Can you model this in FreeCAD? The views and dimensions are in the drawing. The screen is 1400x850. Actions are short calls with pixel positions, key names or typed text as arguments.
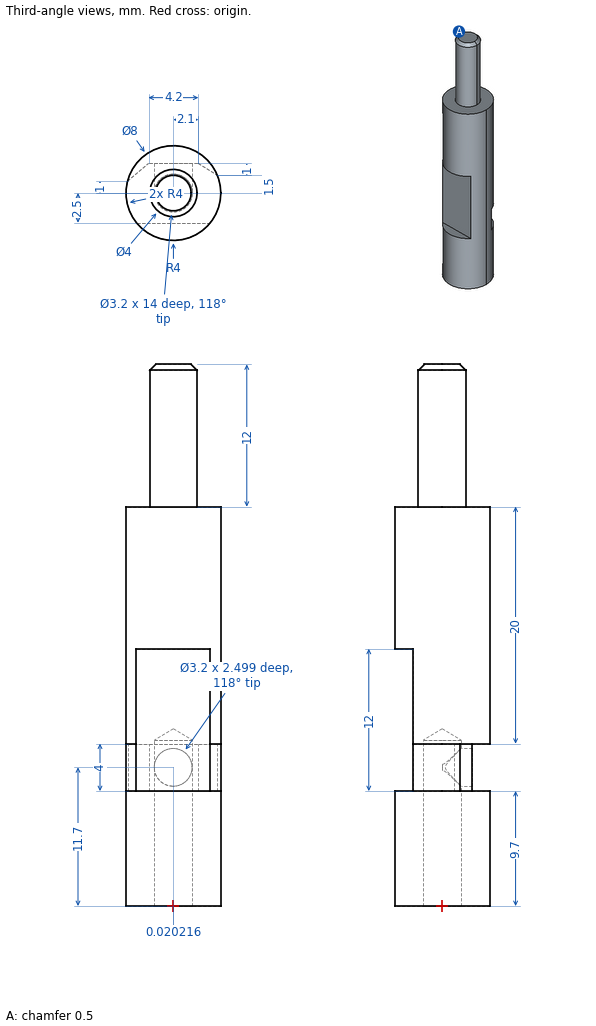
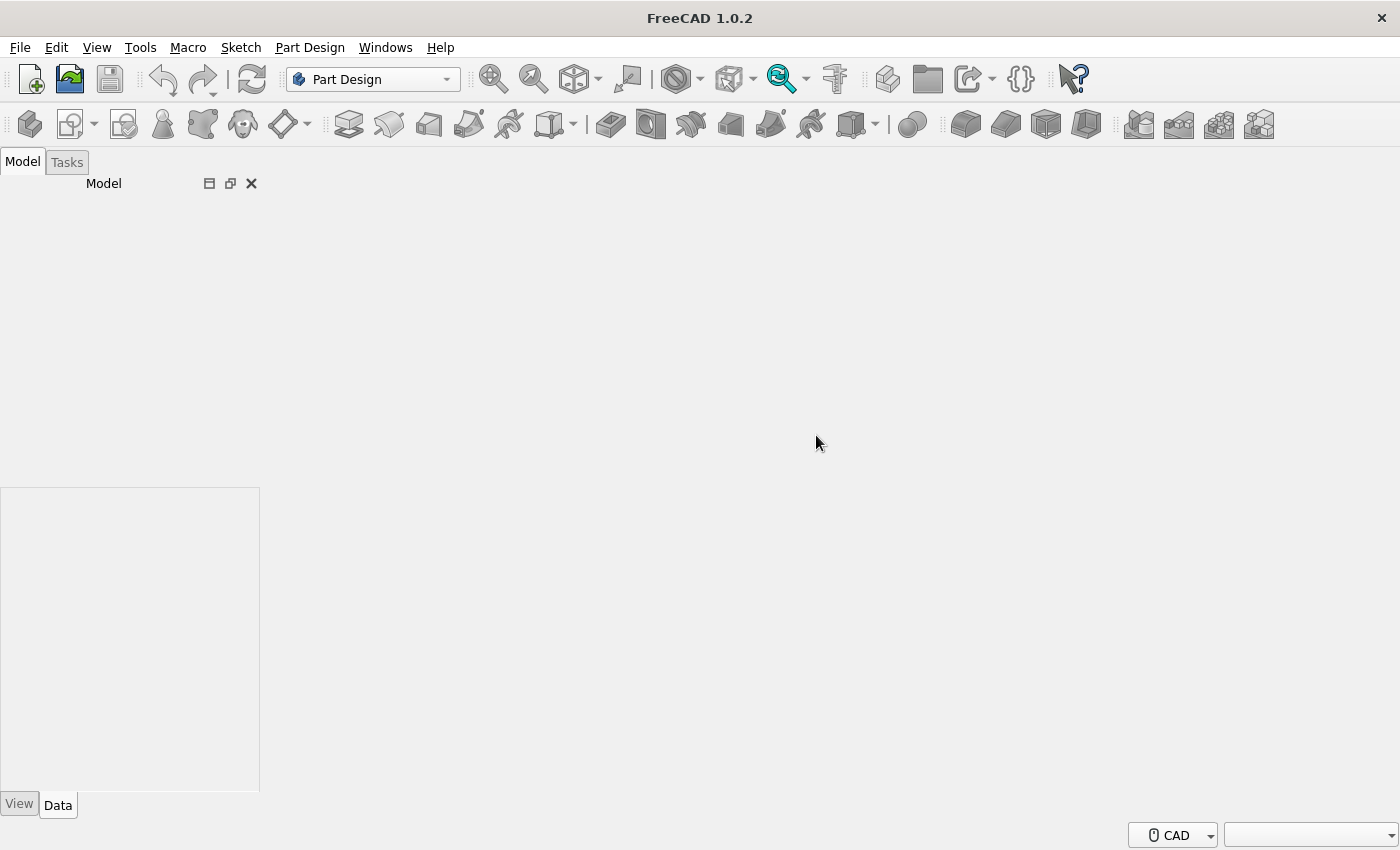
click(30, 80)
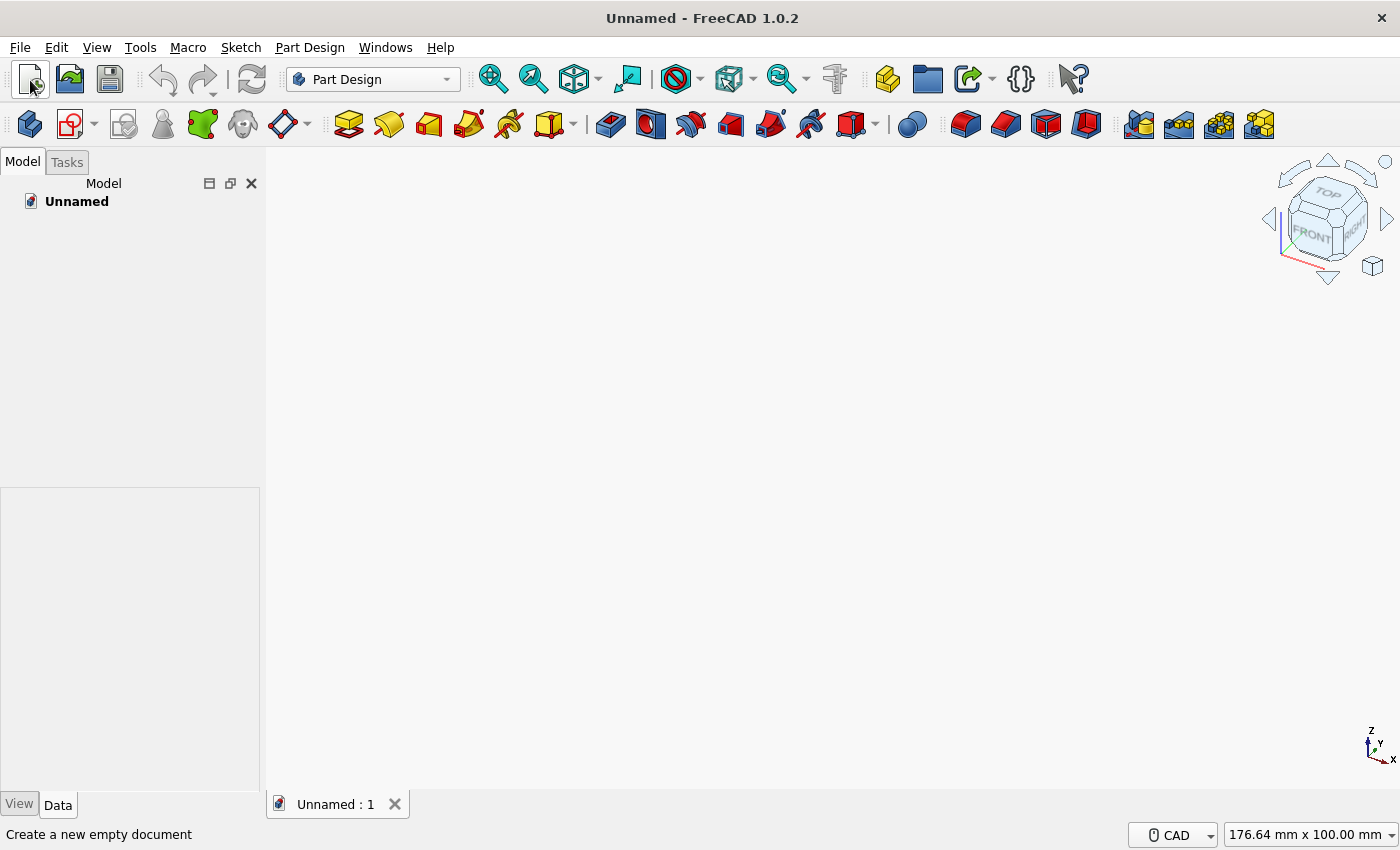
click(70, 124)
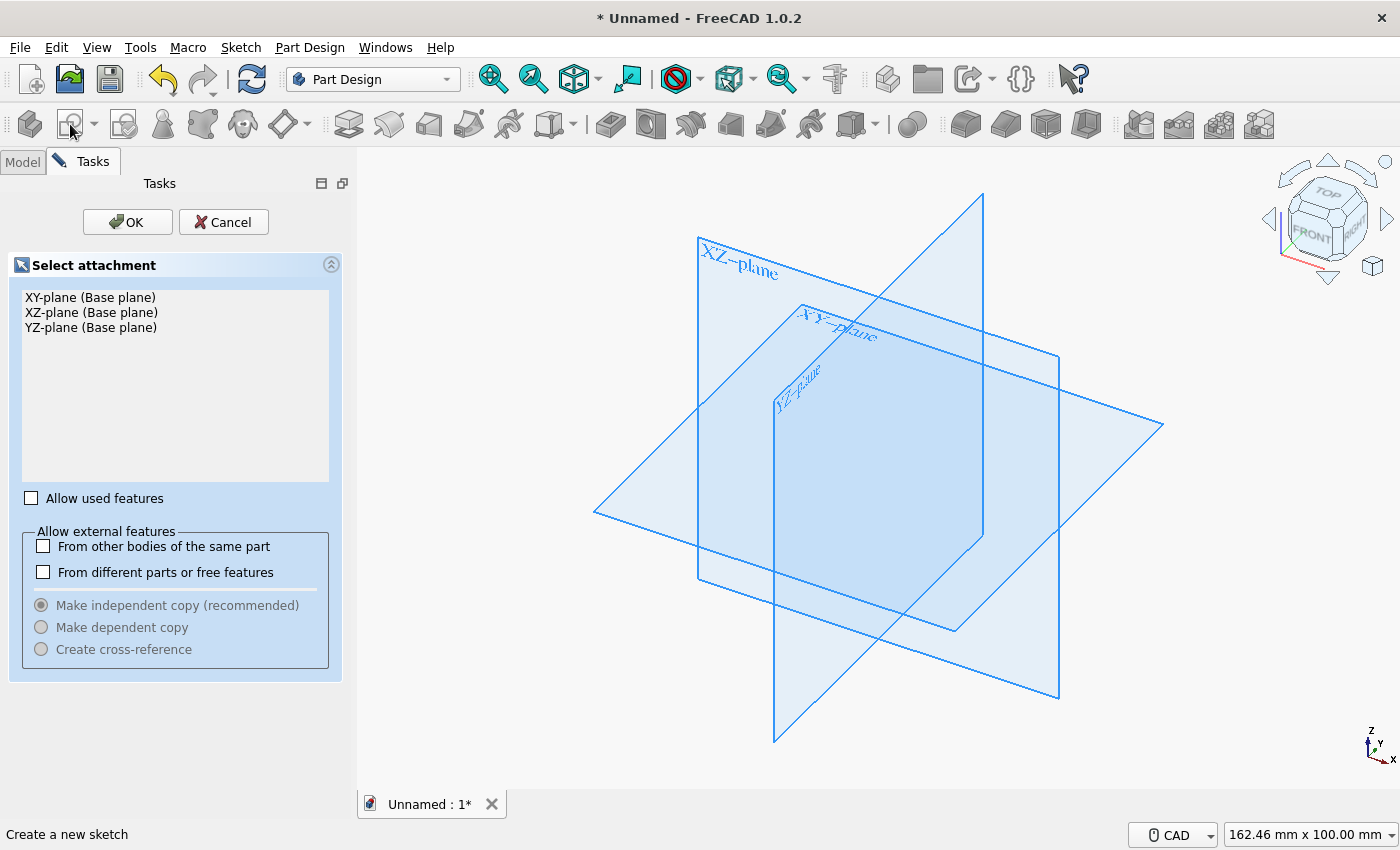
click(82, 298)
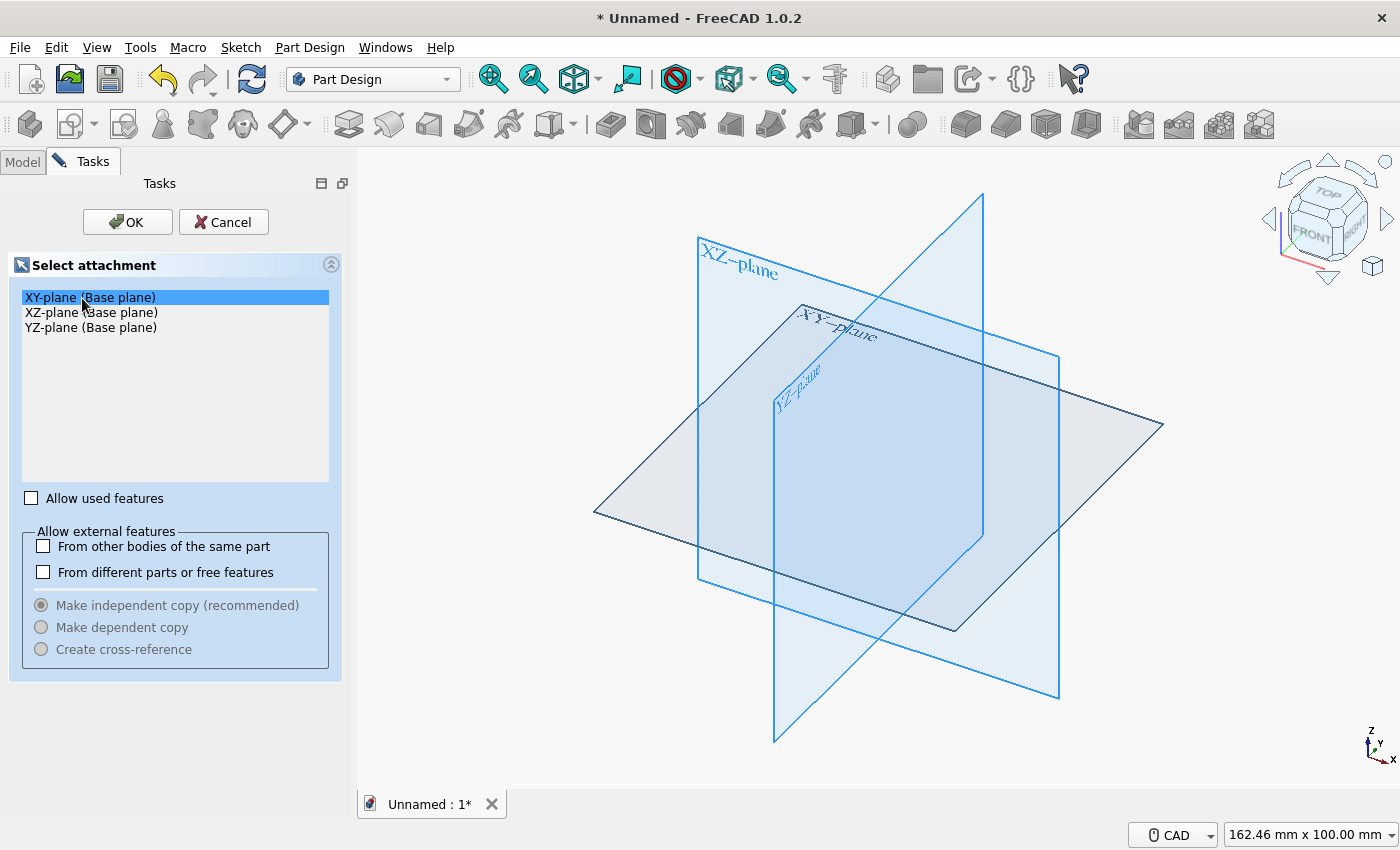
click(128, 222)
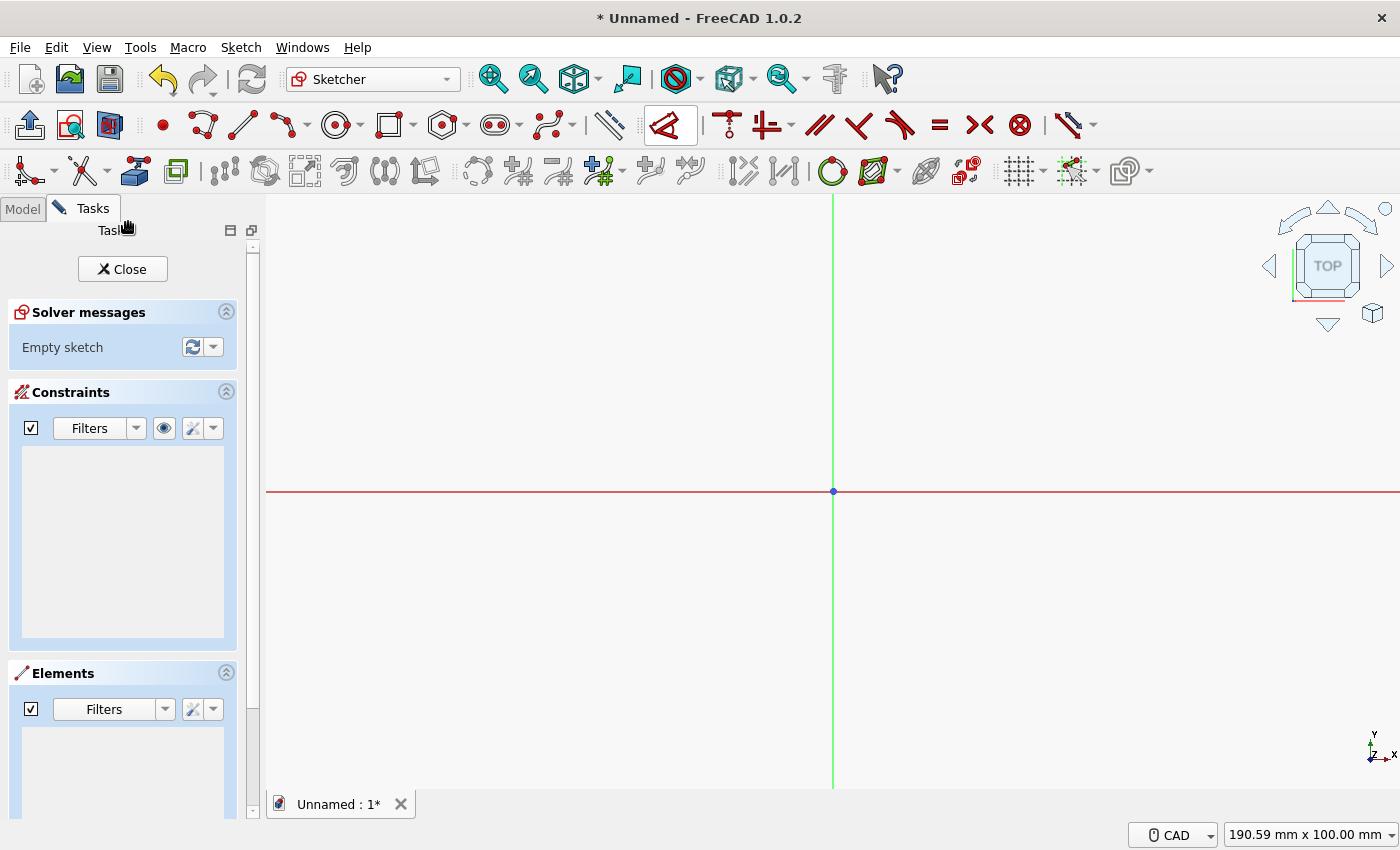
scroll(844, 492, up, 10)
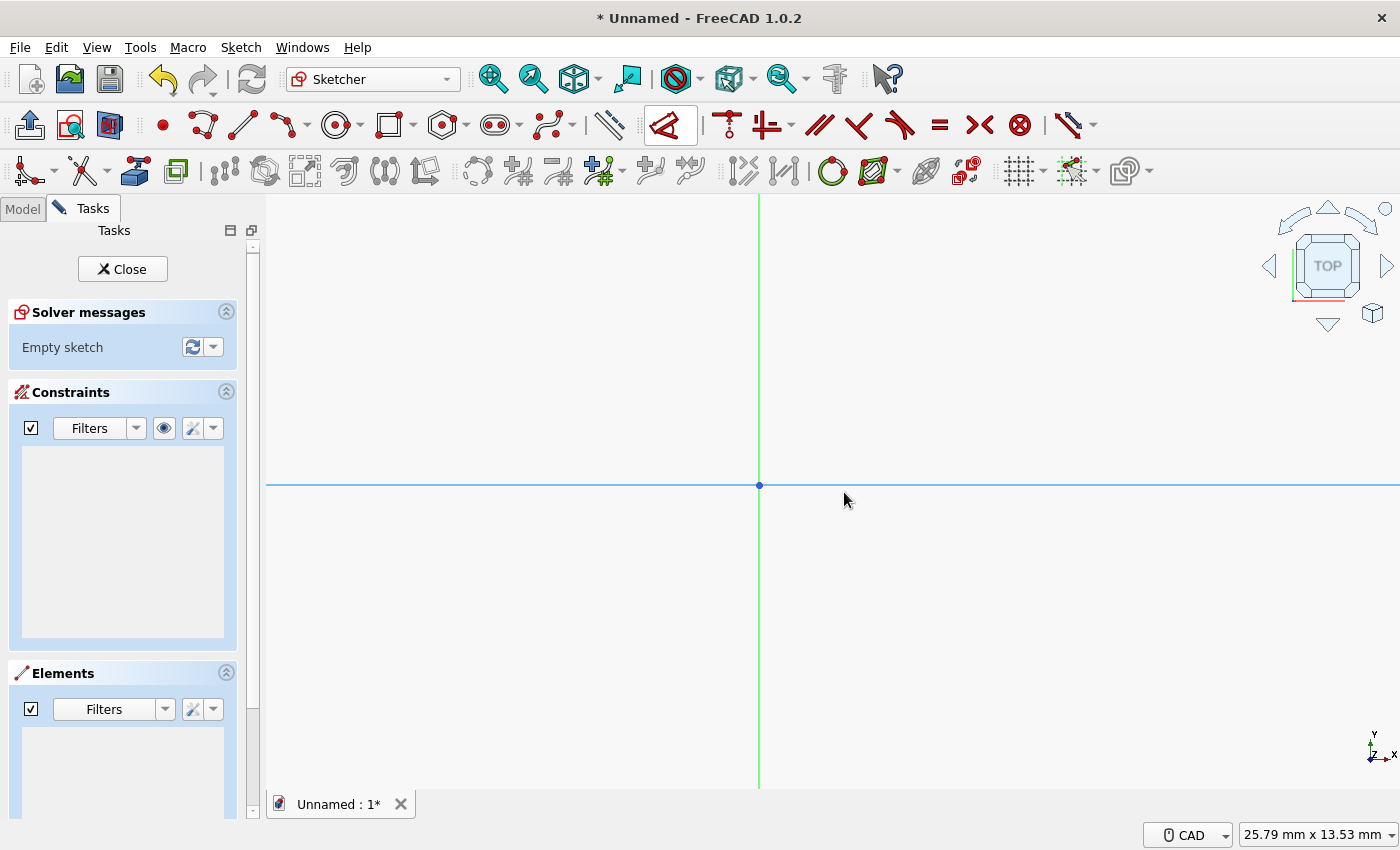
key(g)
key(c)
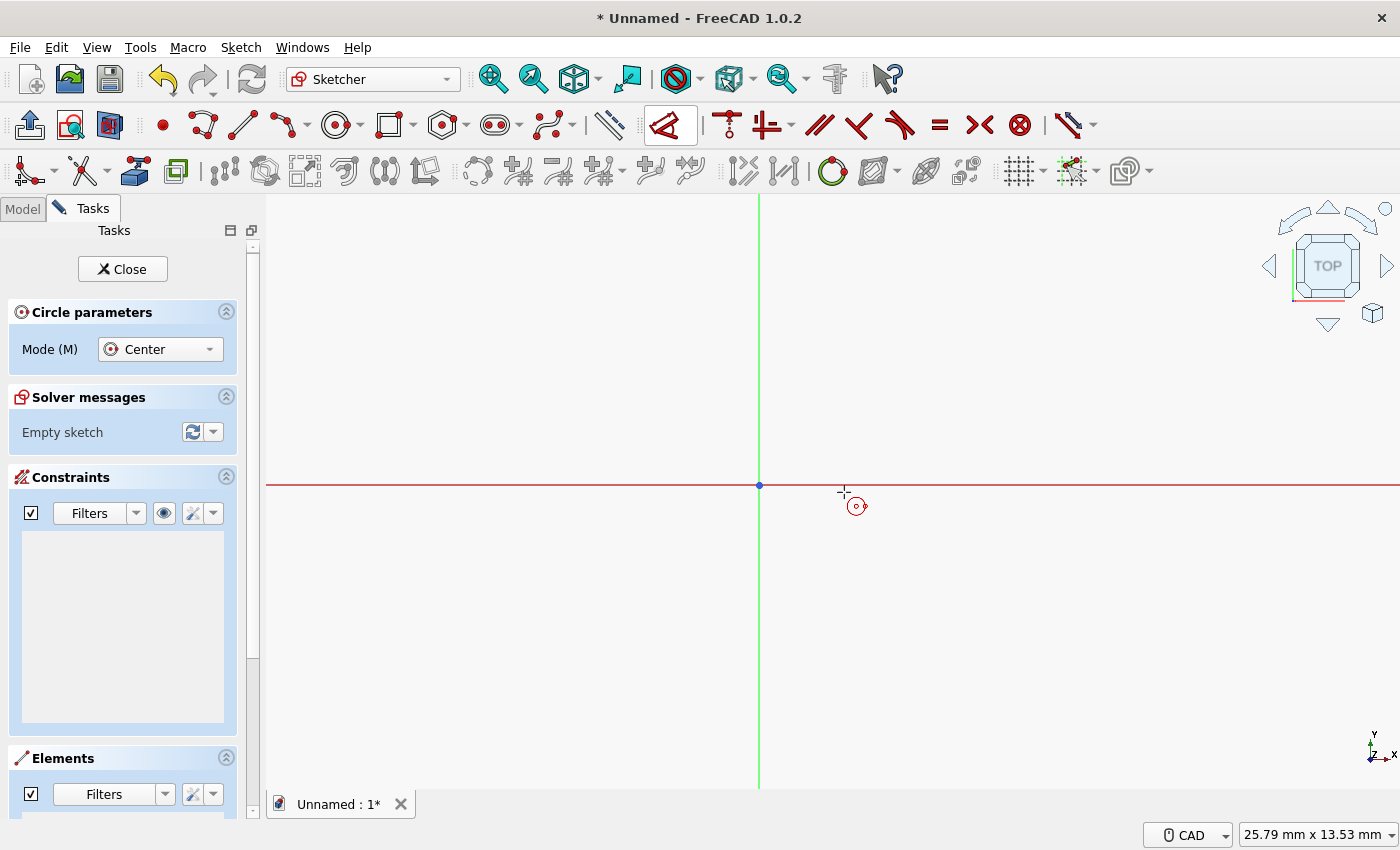
click(759, 485)
click(884, 361)
key(Escape)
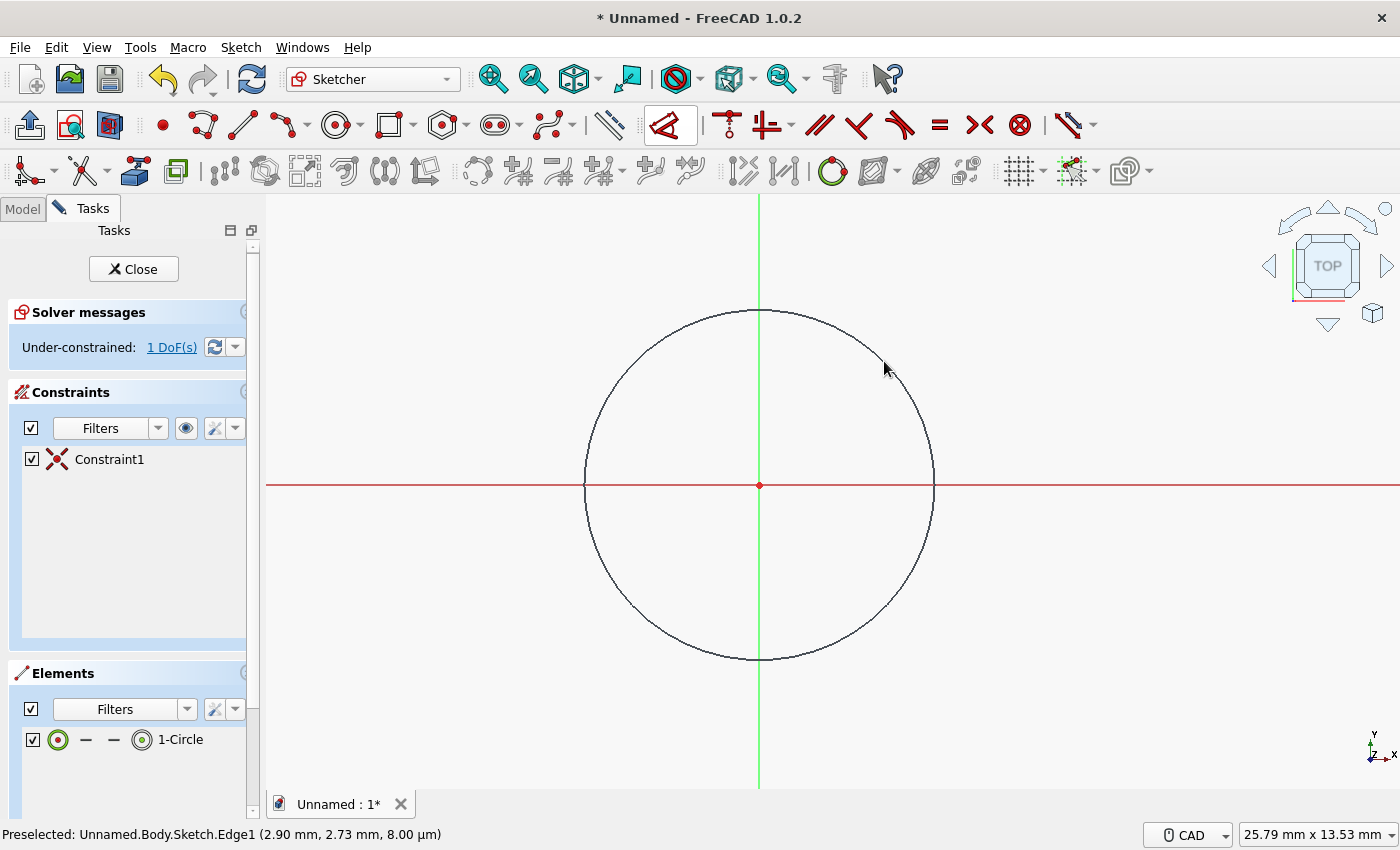
click(664, 126)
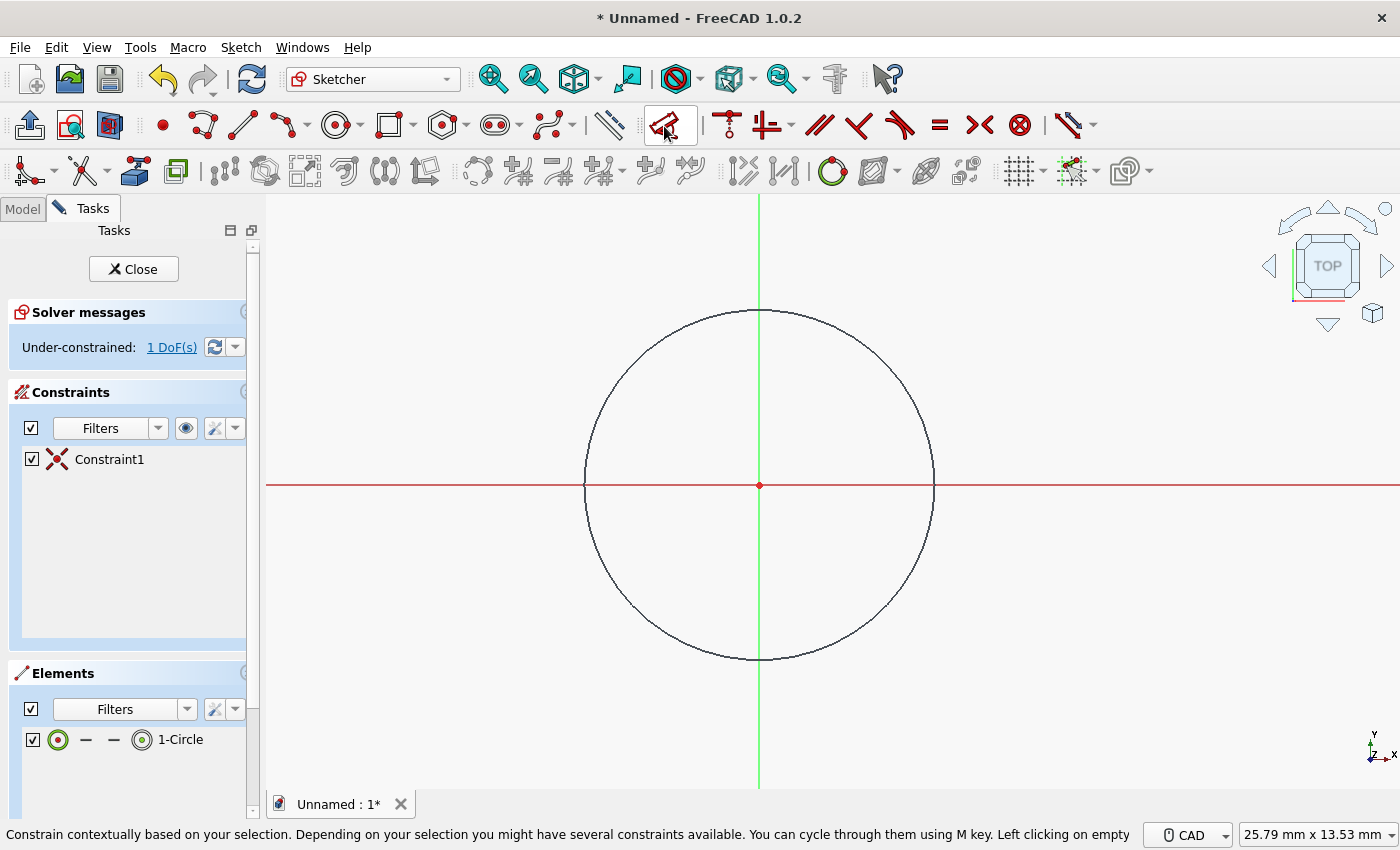
click(883, 361)
click(906, 338)